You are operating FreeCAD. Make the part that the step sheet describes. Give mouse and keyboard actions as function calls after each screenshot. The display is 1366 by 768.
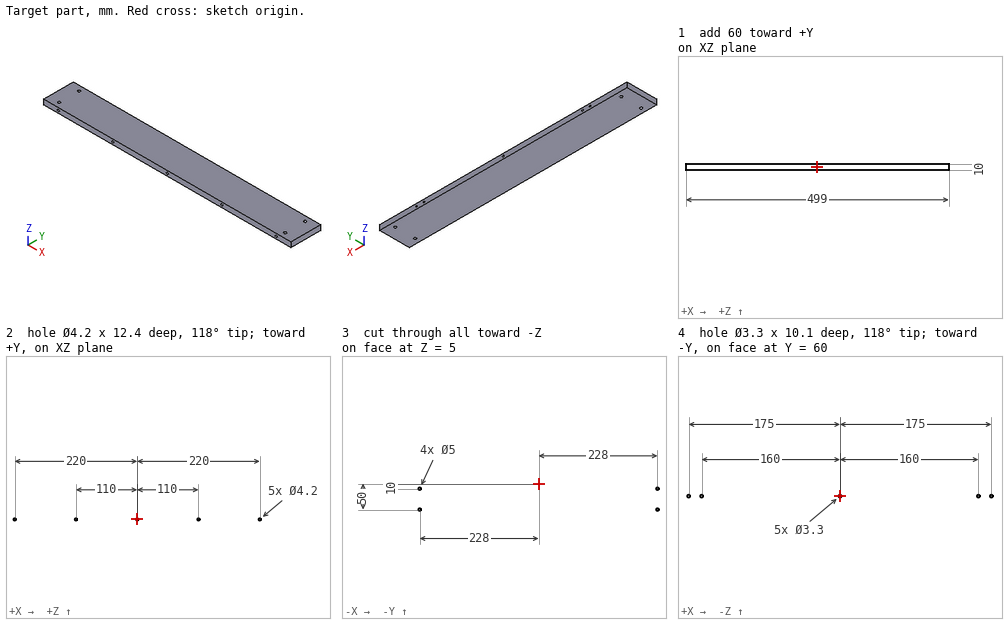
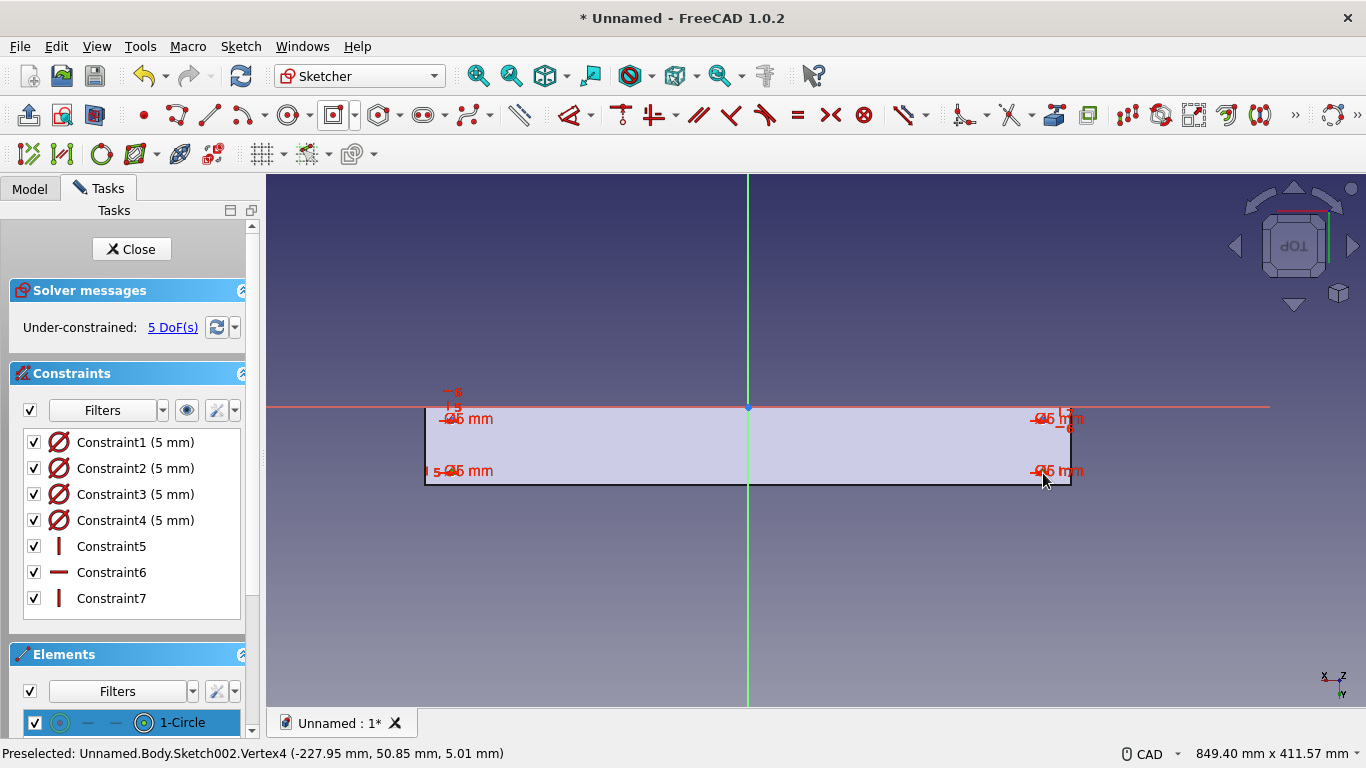
key(h)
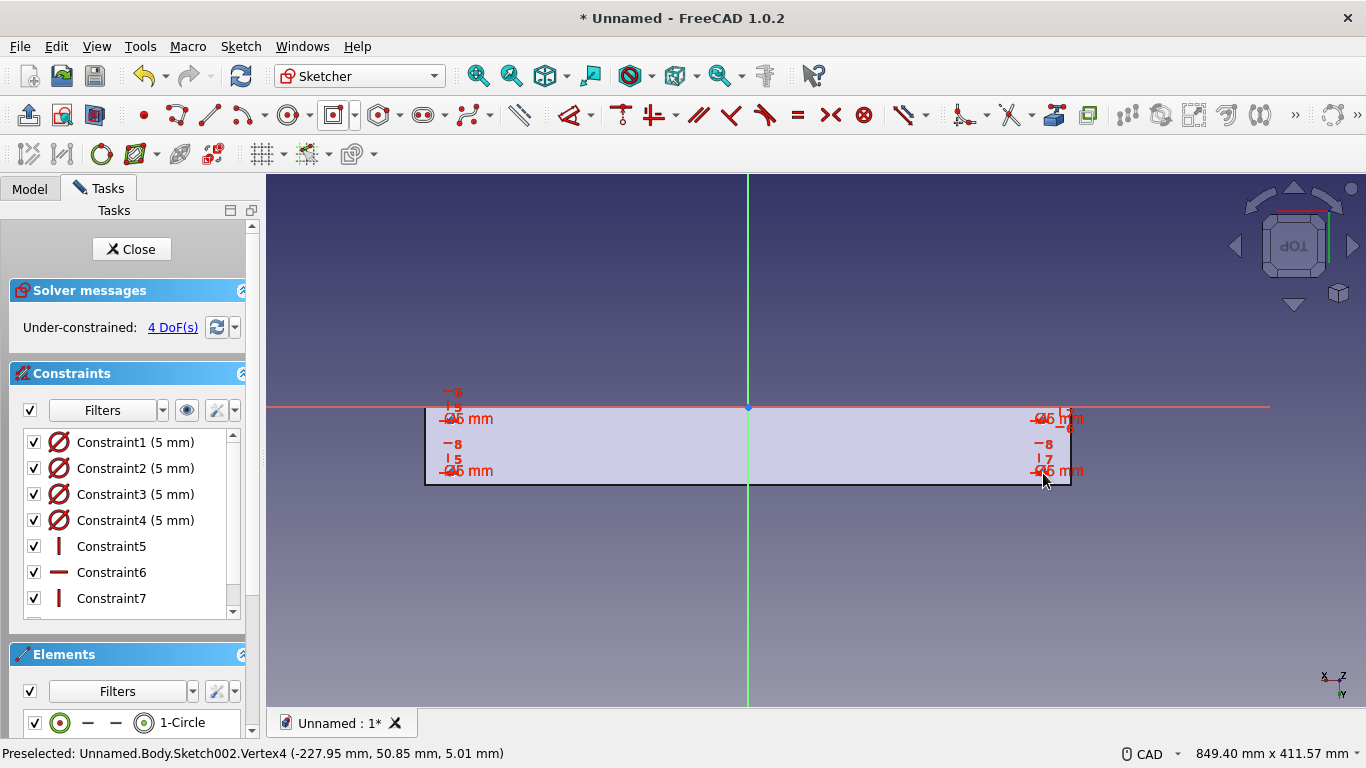
click(568, 116)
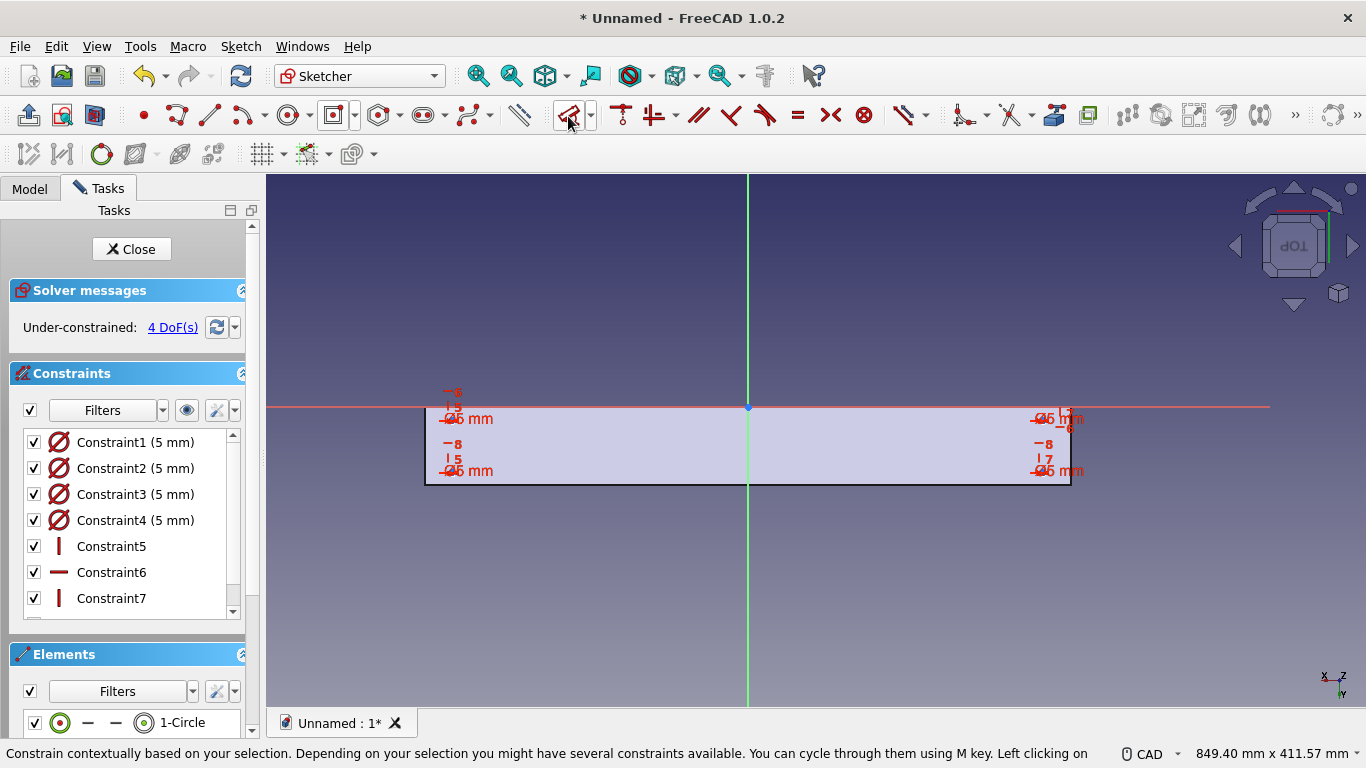
click(453, 473)
click(419, 440)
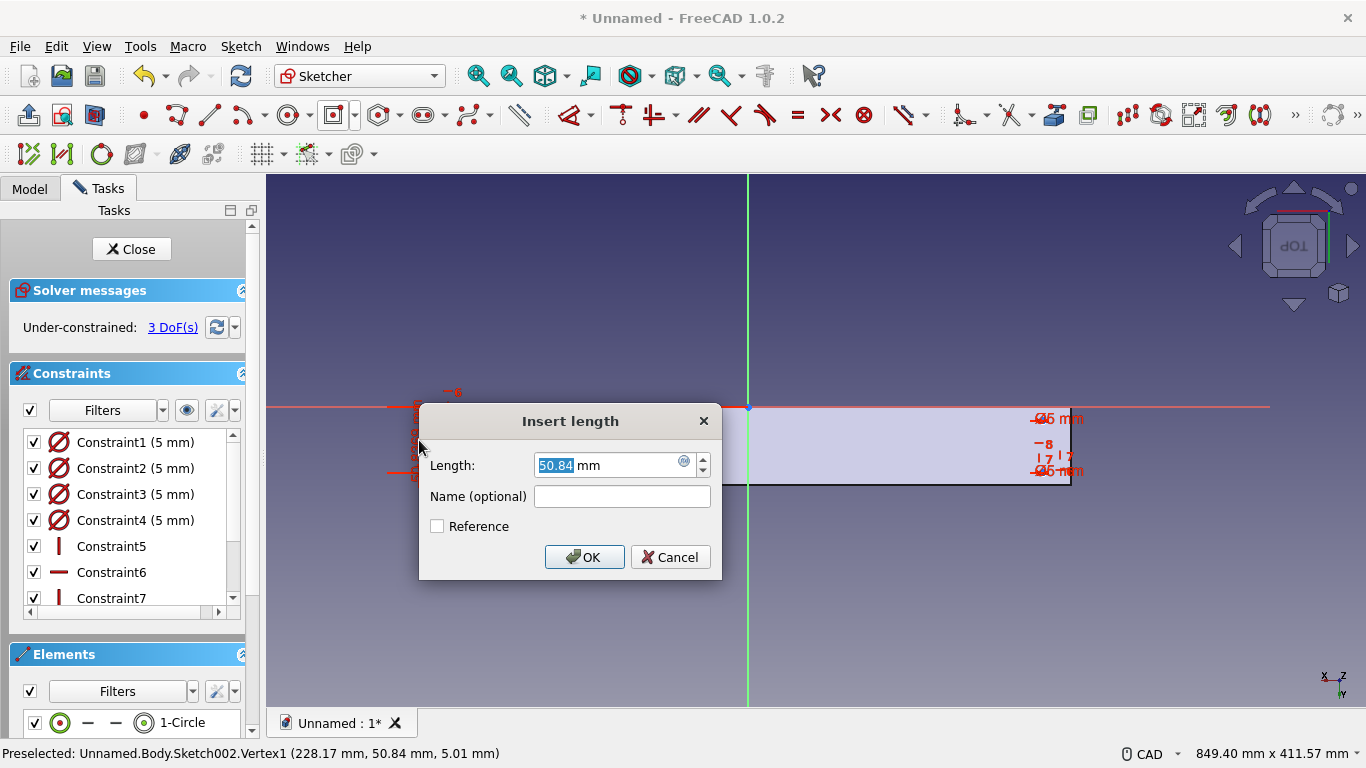
text(50)
key(Return)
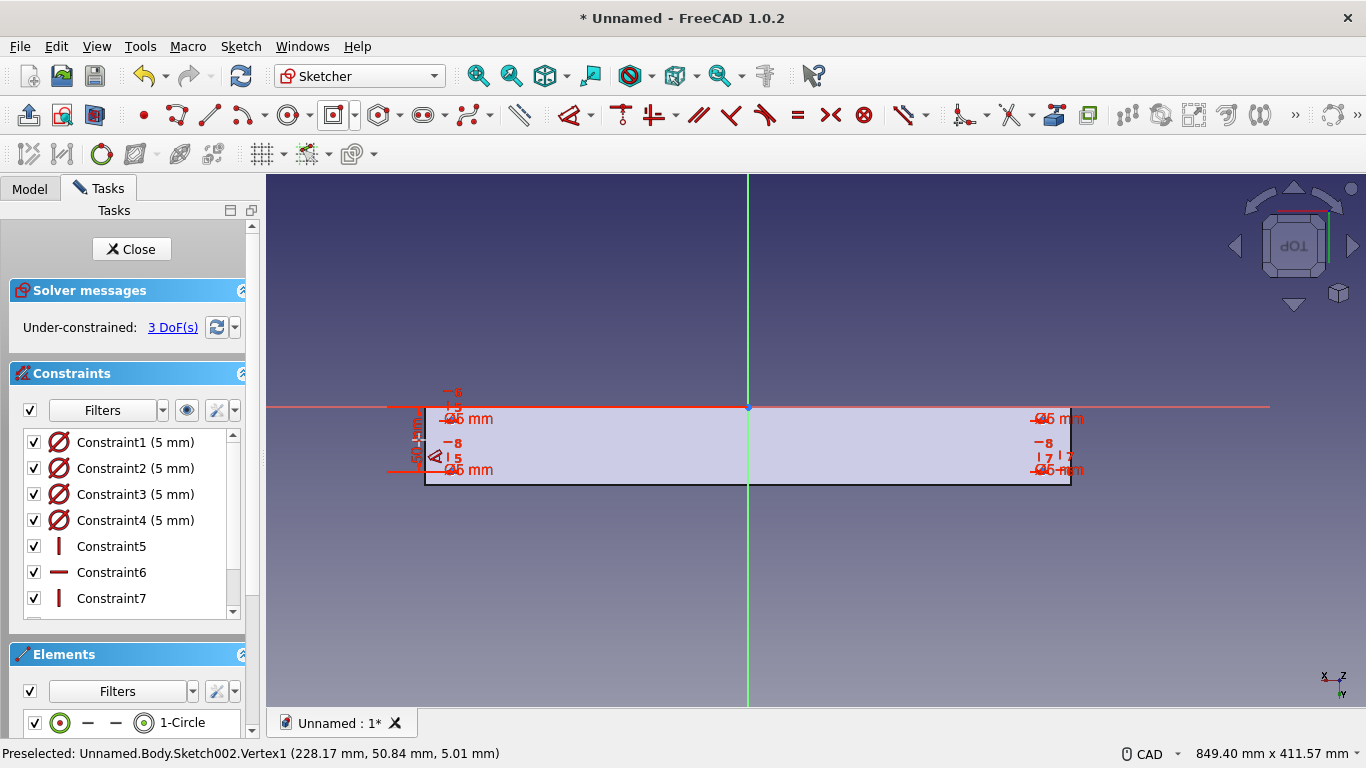
scroll(453, 421, up, 6)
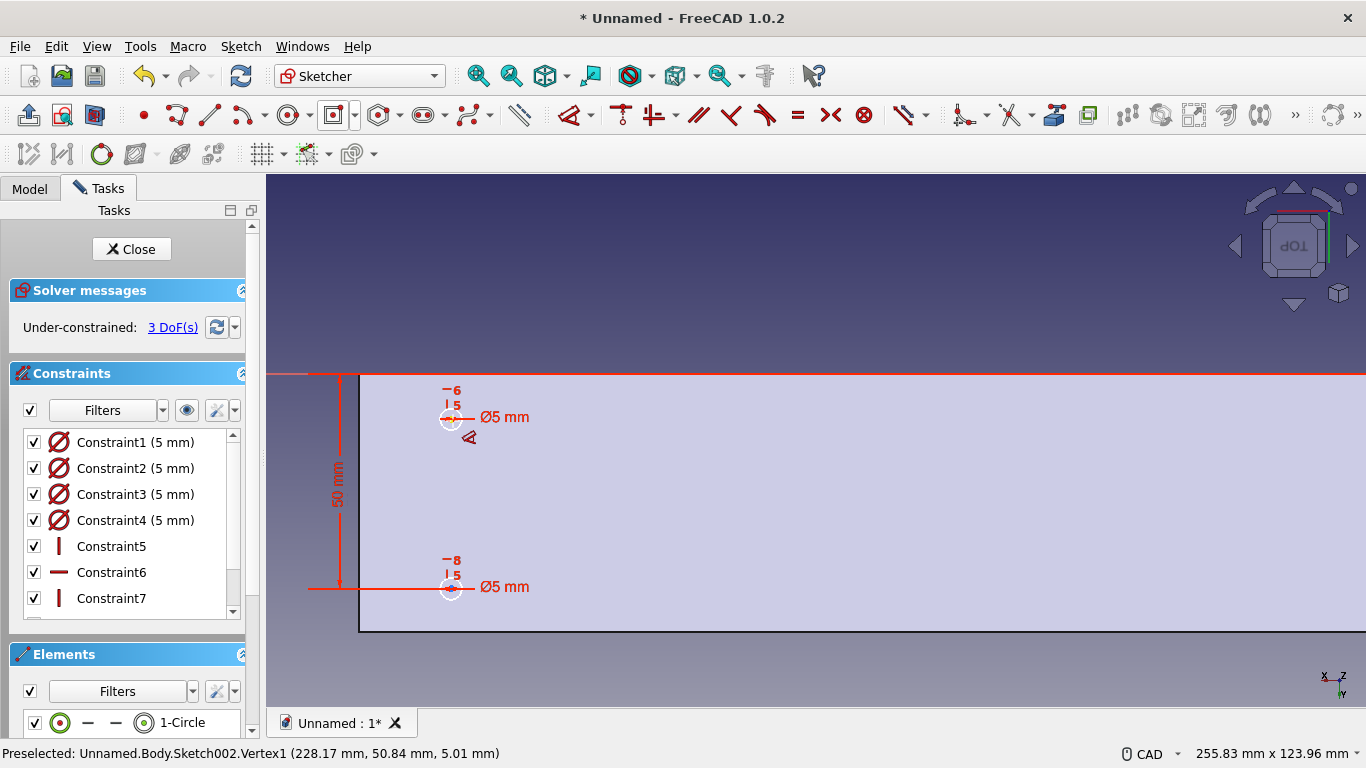
click(451, 419)
click(417, 397)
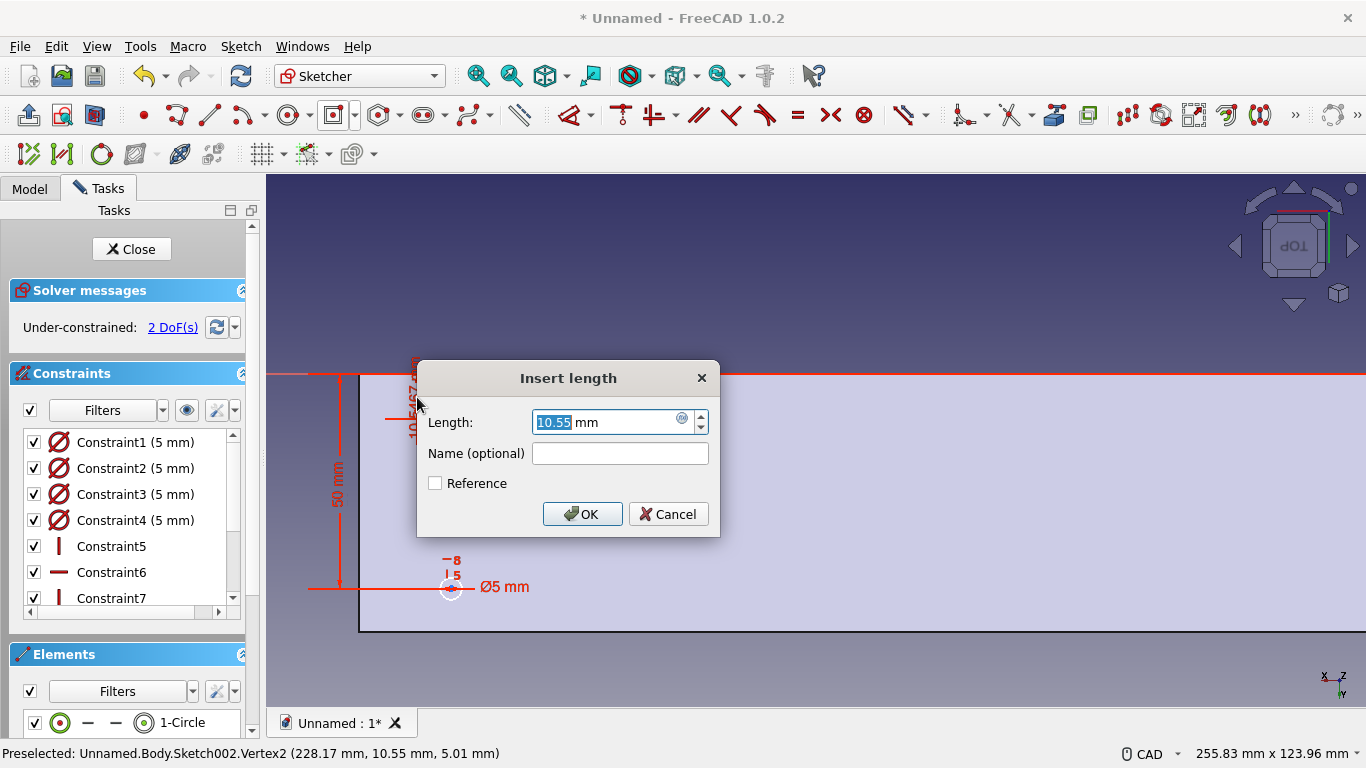
text(10)
key(Return)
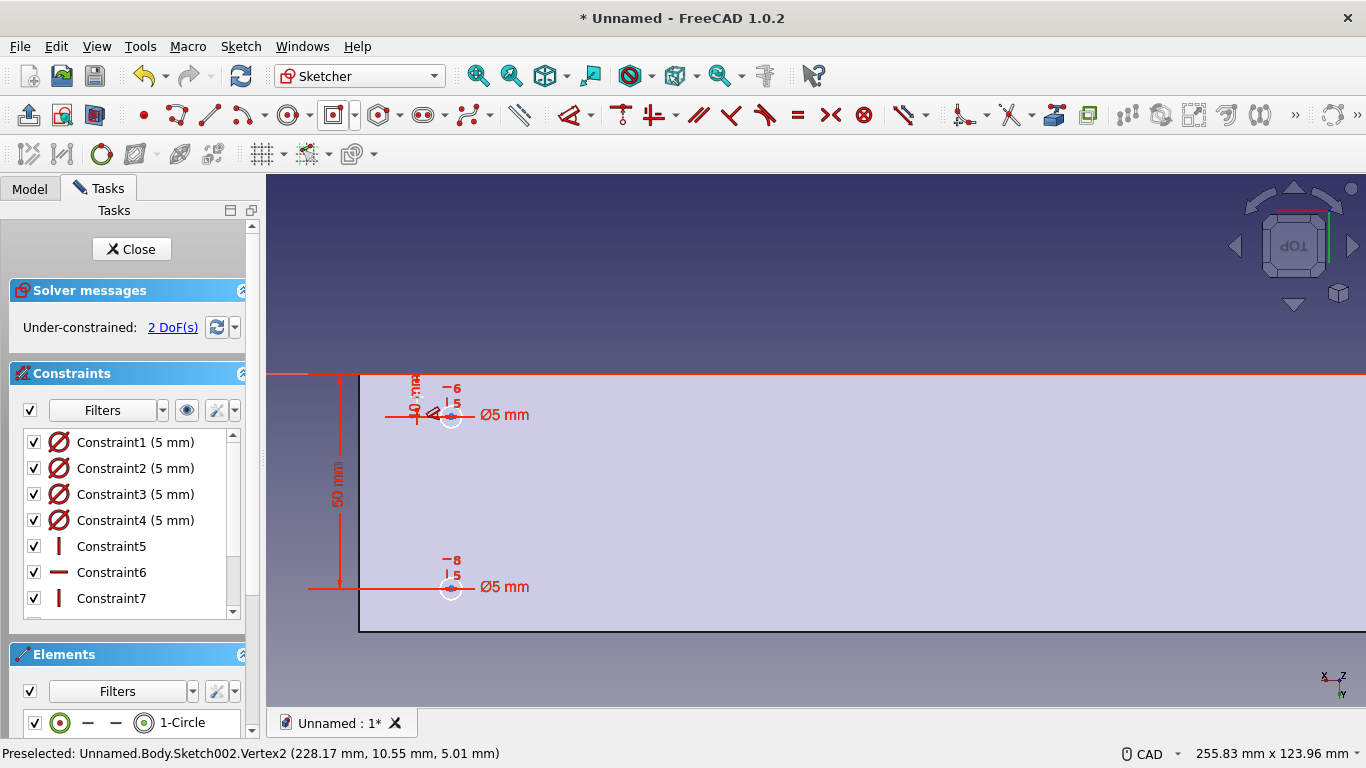
scroll(452, 421, down, 6)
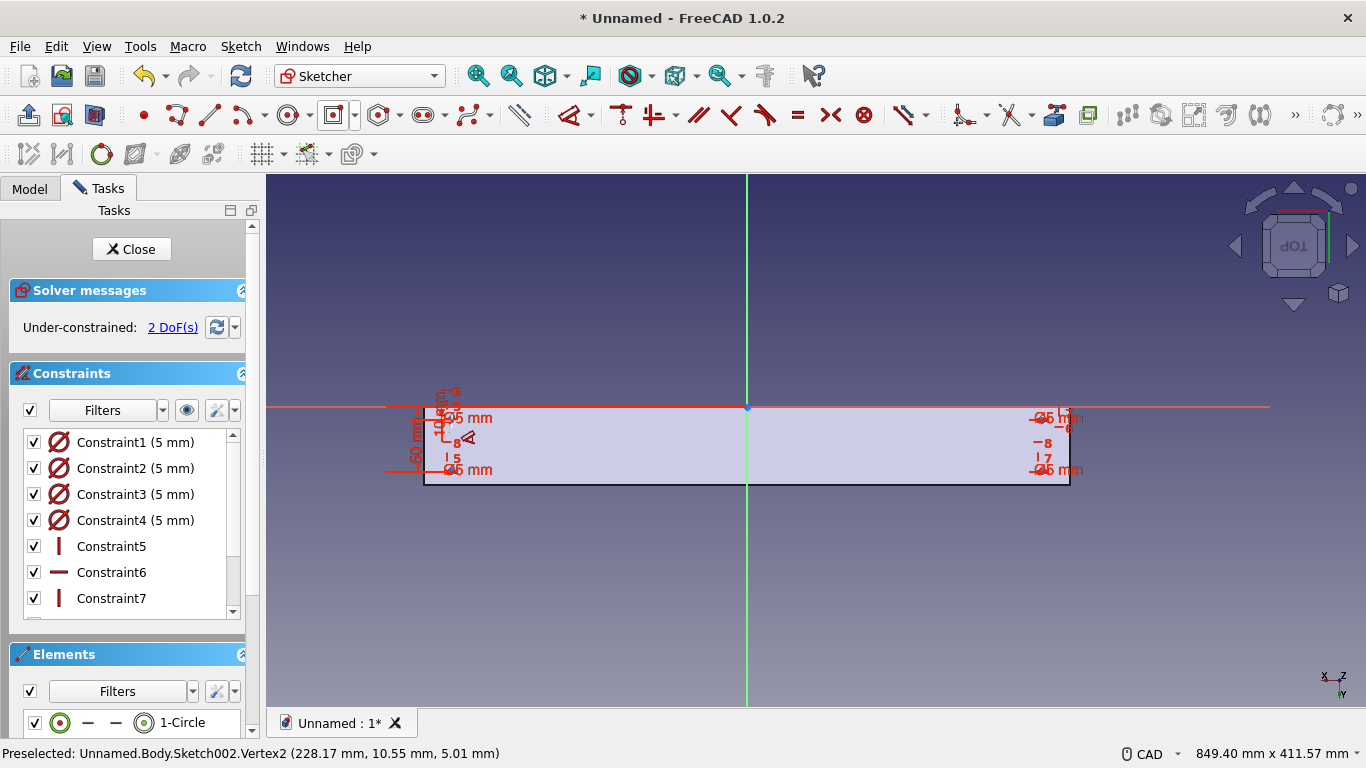
click(452, 472)
click(600, 373)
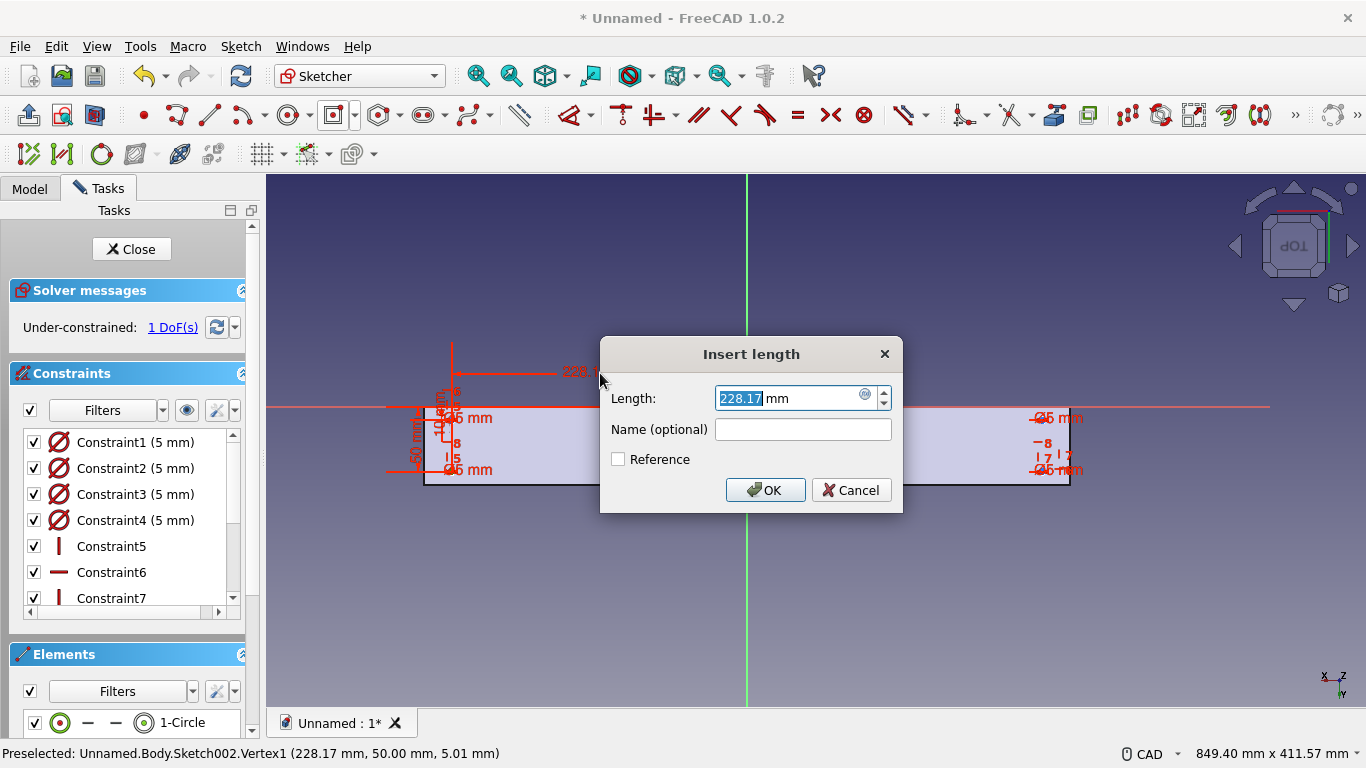
text(228)
key(Return)